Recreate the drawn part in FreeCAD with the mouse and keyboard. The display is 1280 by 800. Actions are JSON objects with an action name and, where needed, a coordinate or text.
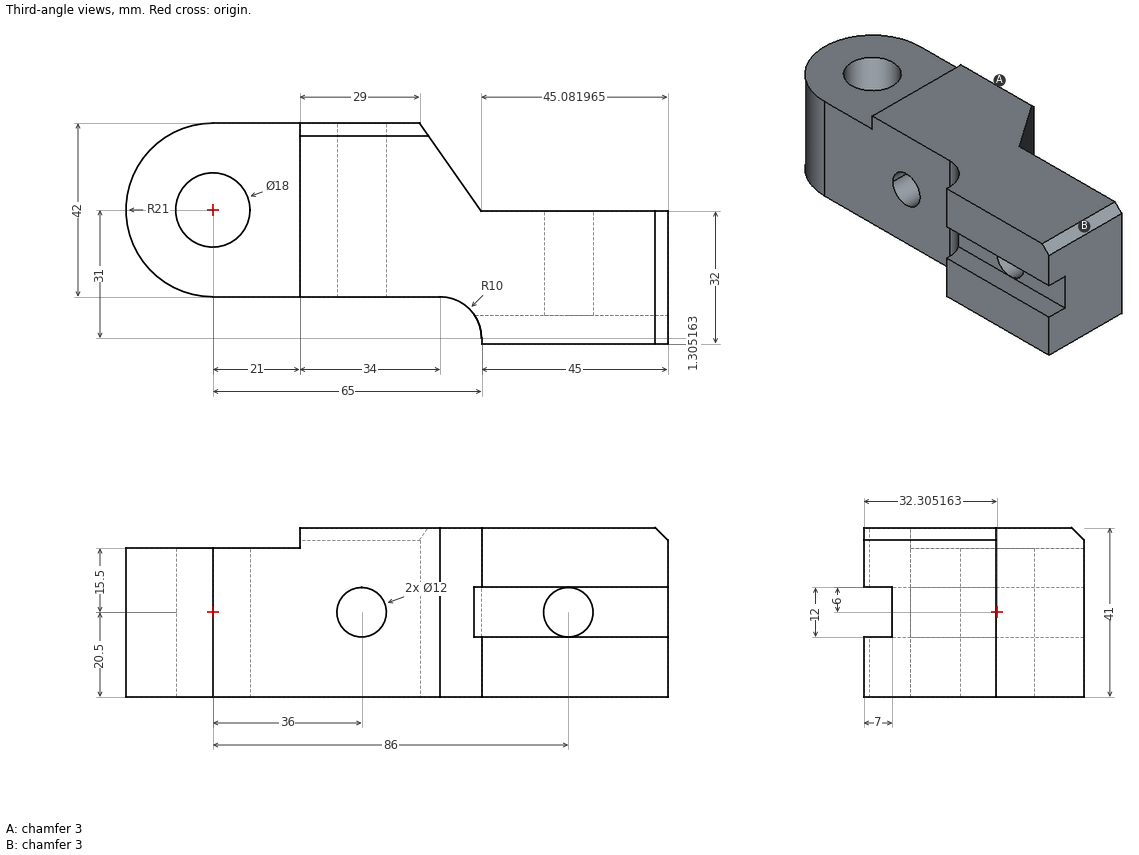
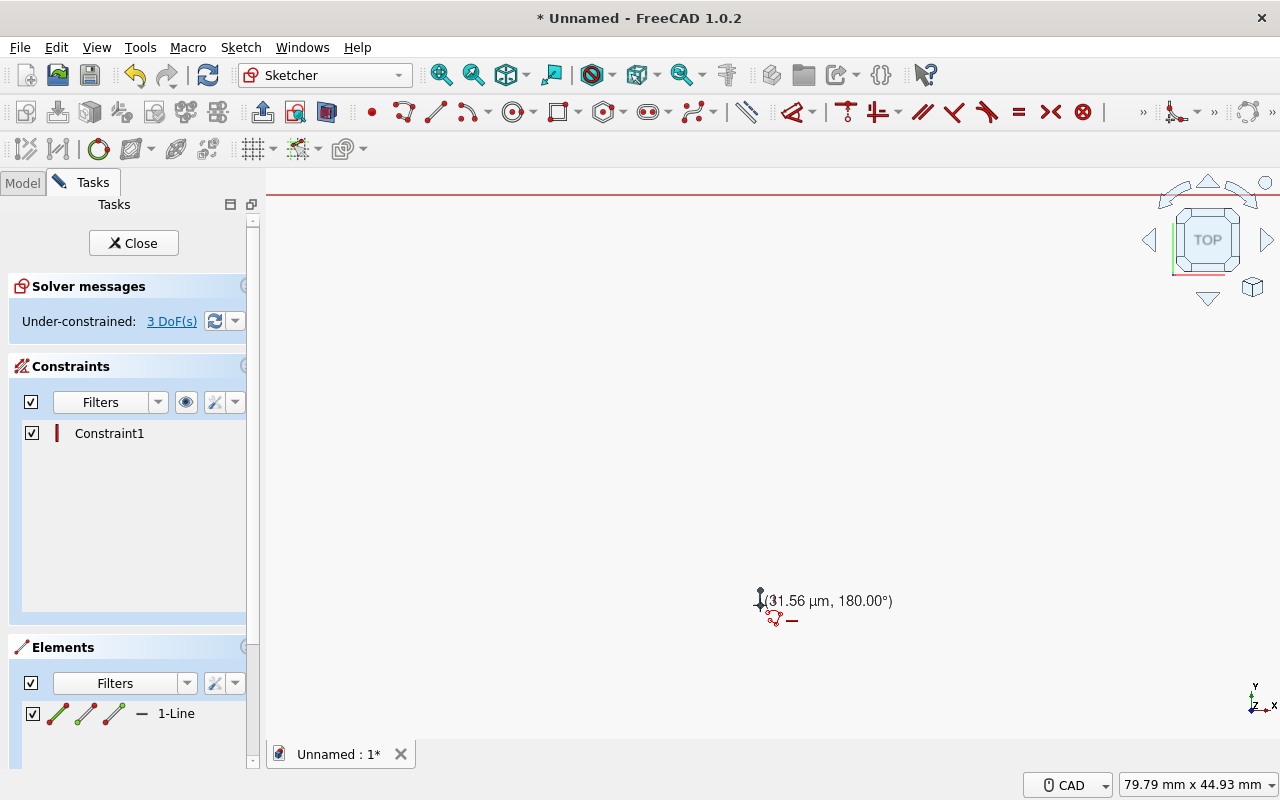
{"action": "scroll", "coordinate": [762, 606], "scroll_direction": "down", "scroll_amount": 4}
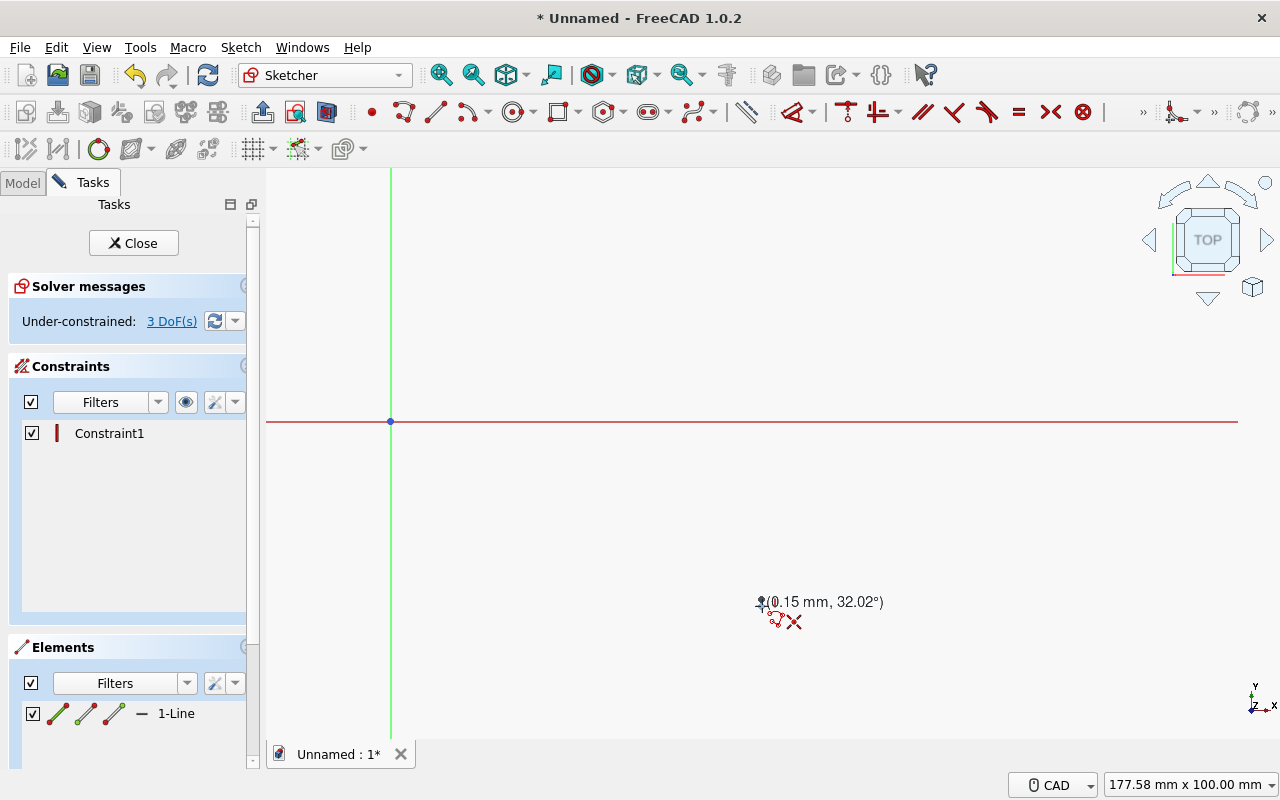
{"action": "left_click", "coordinate": [1019, 606]}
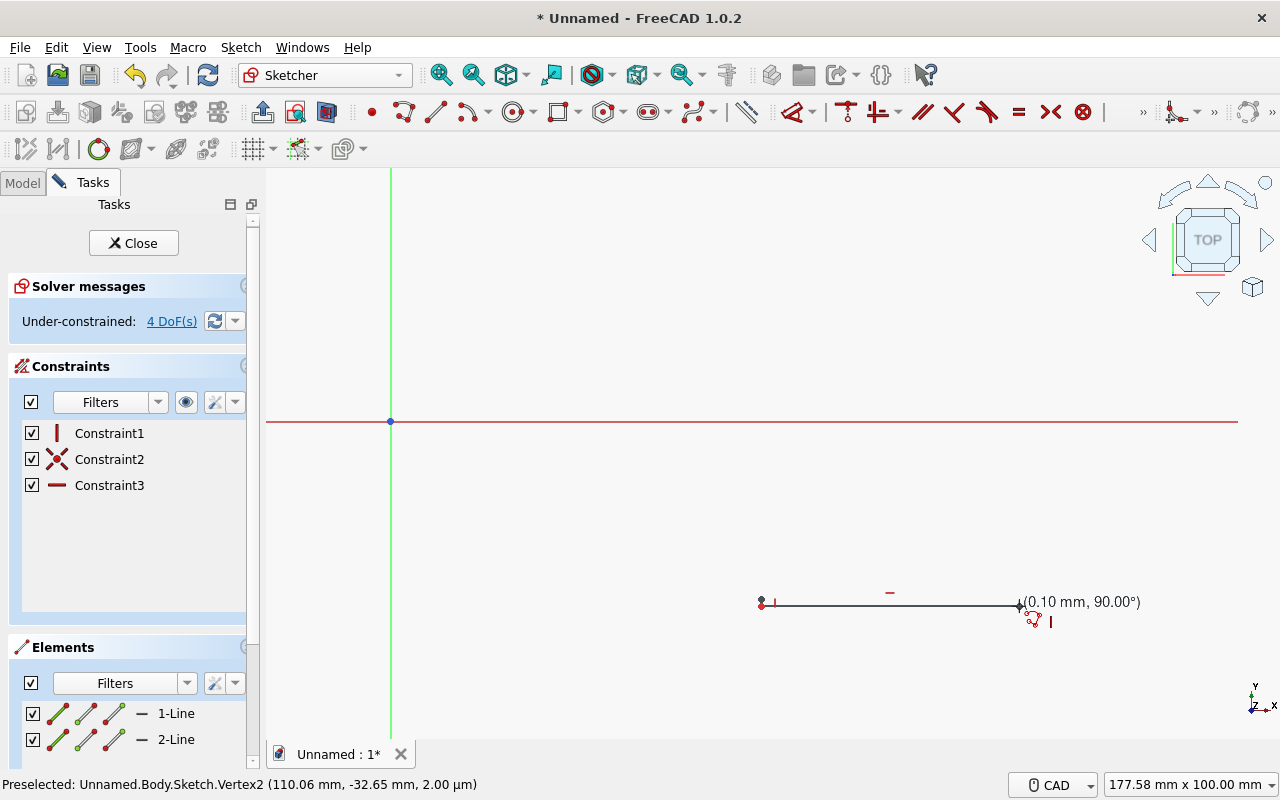
{"action": "scroll", "coordinate": [1019, 423], "scroll_direction": "up", "scroll_amount": 12}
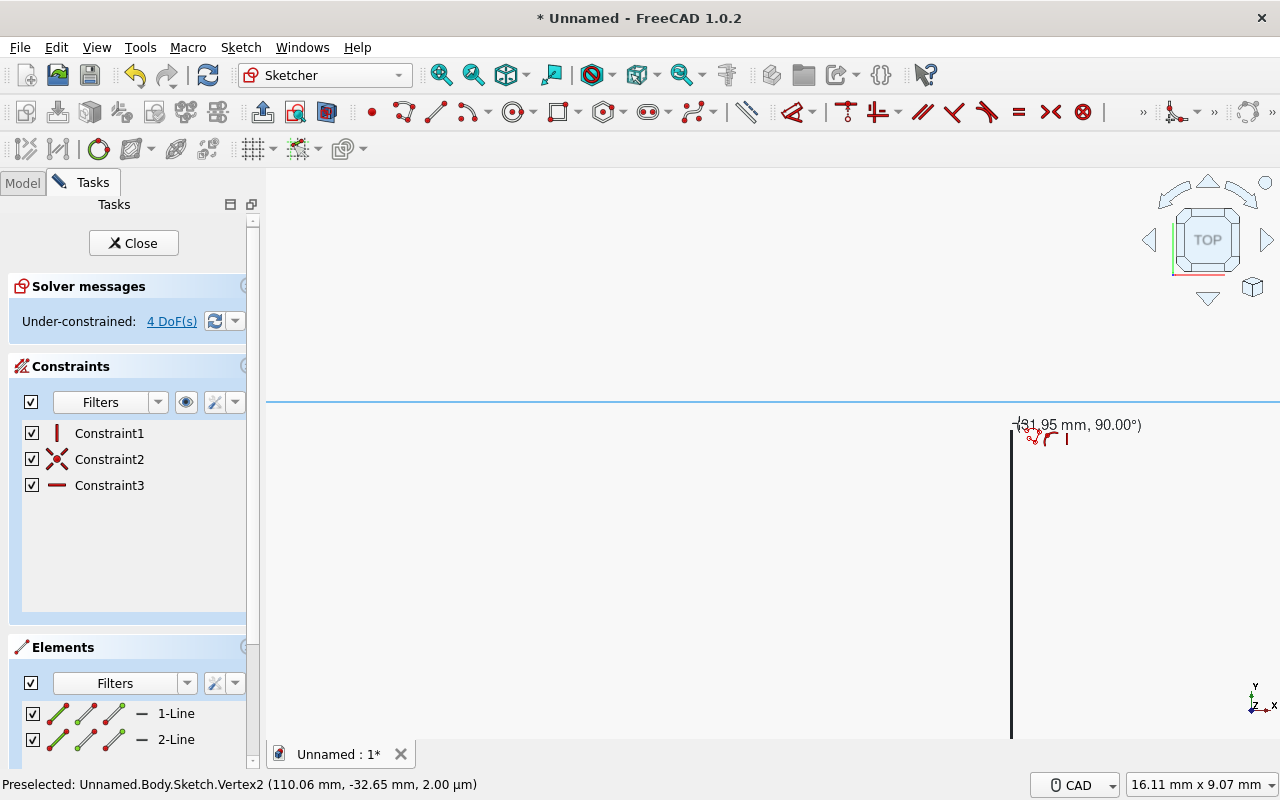
{"action": "left_click", "coordinate": [1012, 422]}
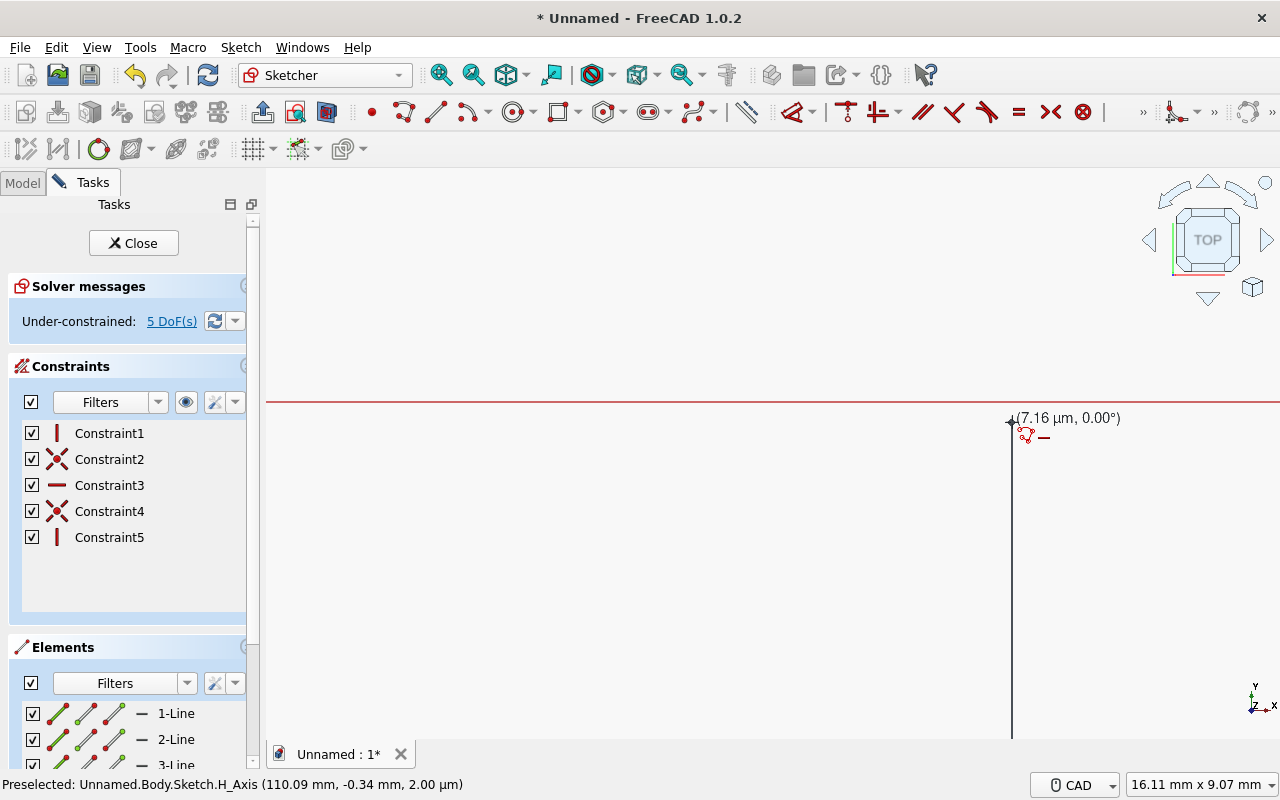
{"action": "scroll", "coordinate": [1020, 423], "scroll_direction": "down", "scroll_amount": 12}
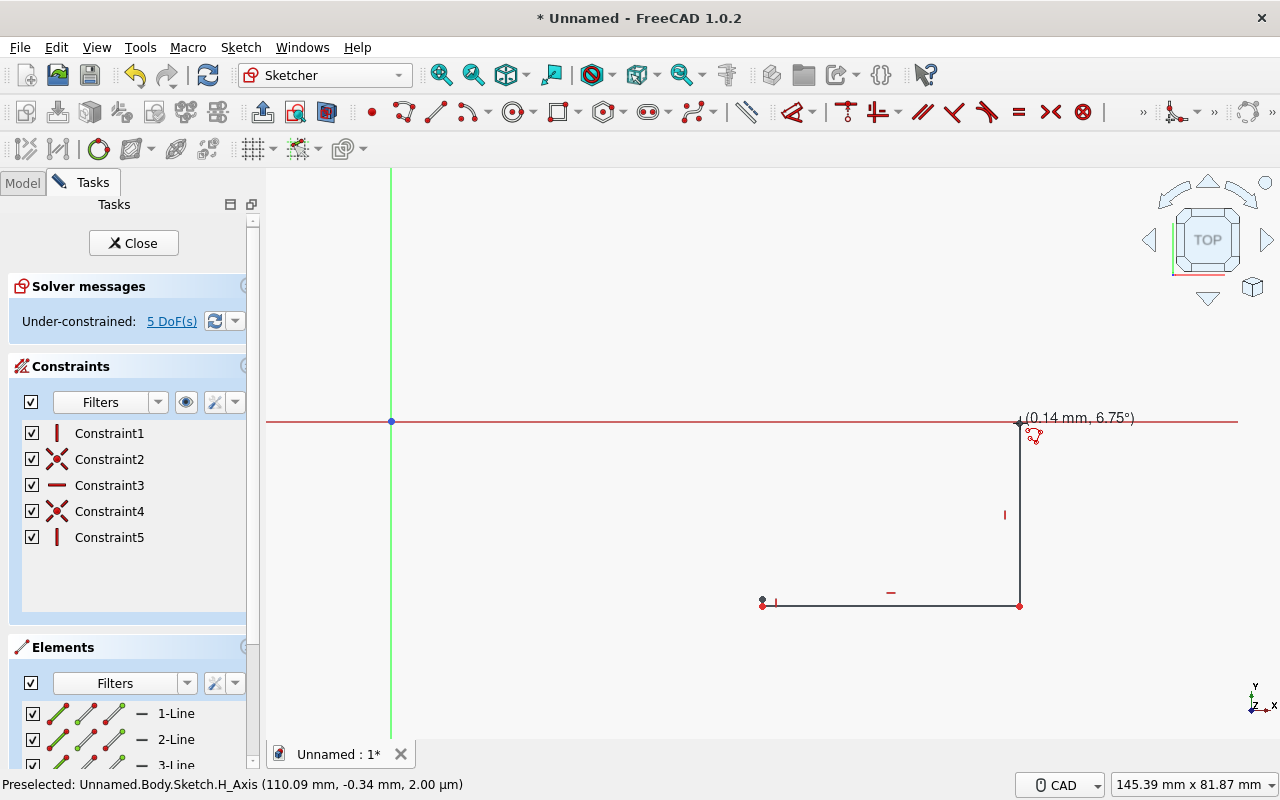
{"action": "scroll", "coordinate": [762, 423], "scroll_direction": "up", "scroll_amount": 12}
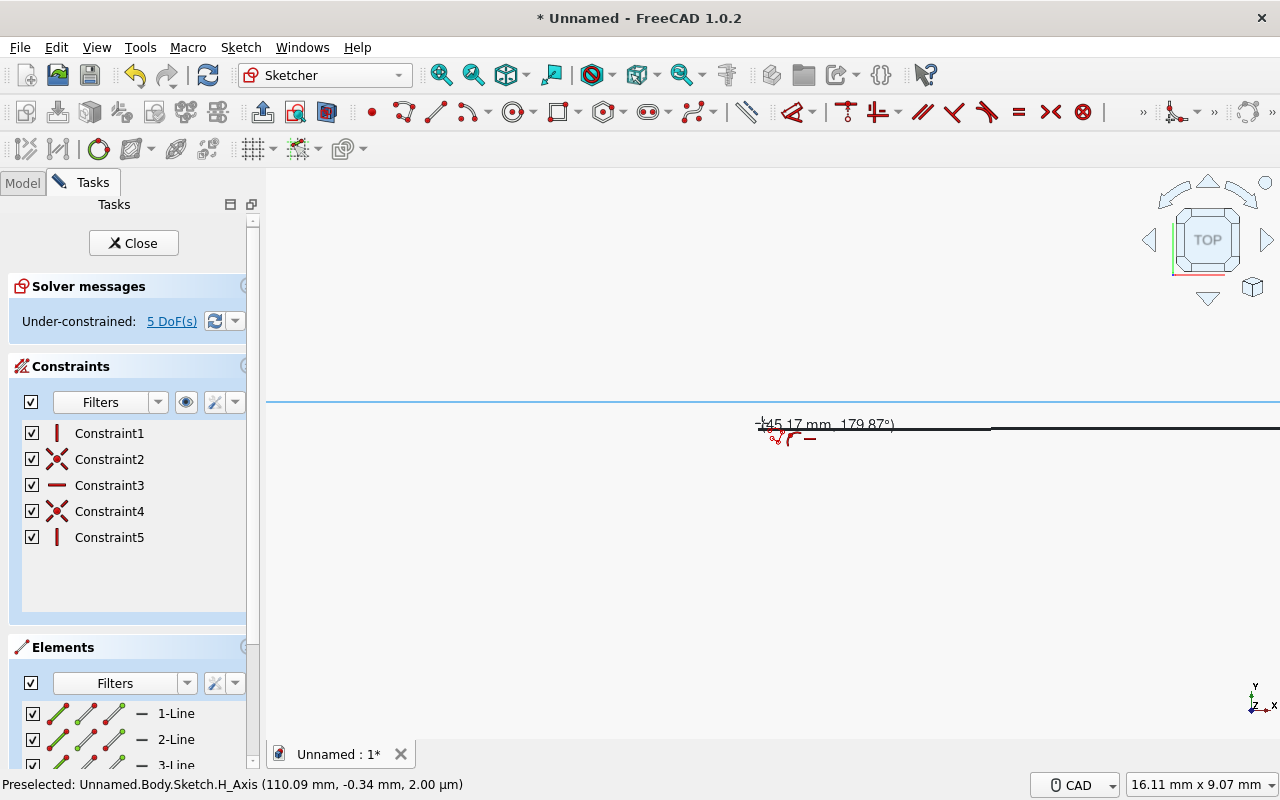
{"action": "left_click", "coordinate": [758, 422]}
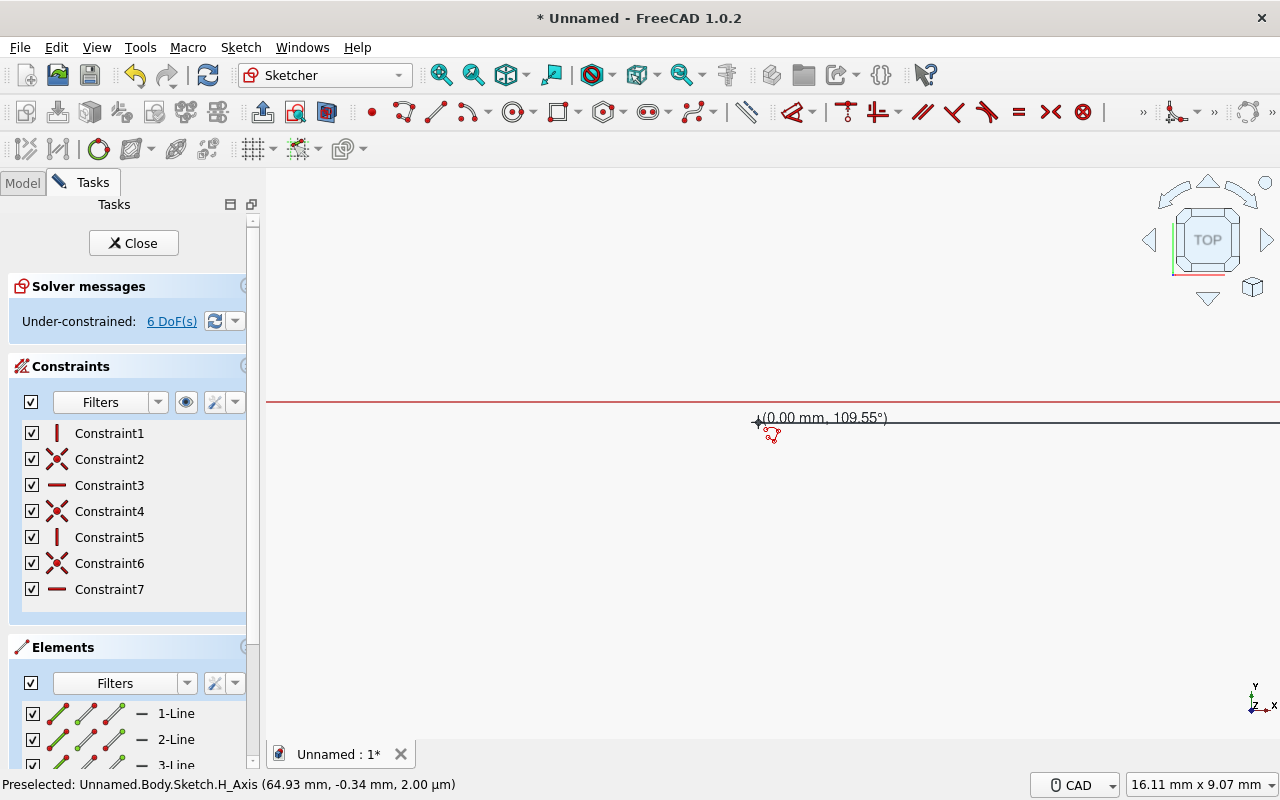
{"action": "scroll", "coordinate": [761, 423], "scroll_direction": "down", "scroll_amount": 12}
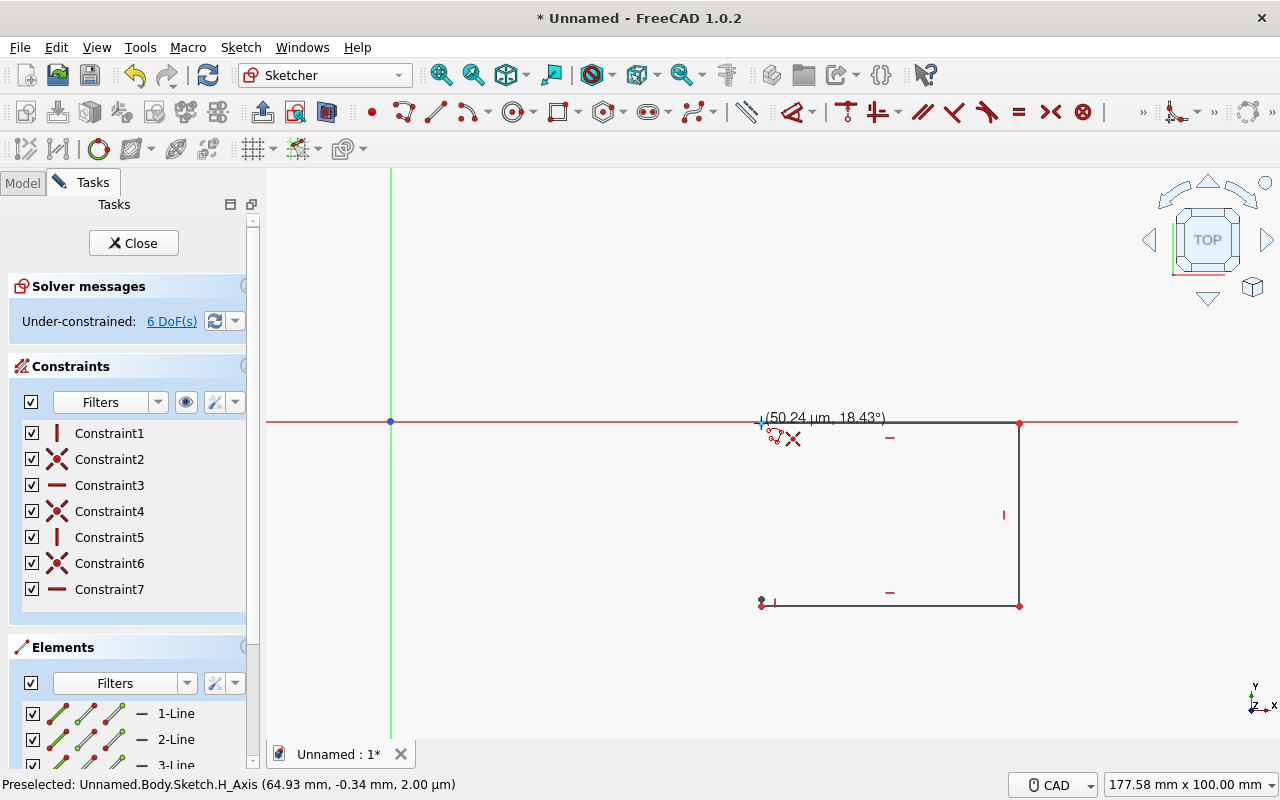
{"action": "left_click", "coordinate": [676, 302]}
{"action": "left_click", "coordinate": [510, 302]}
{"action": "left_click", "coordinate": [510, 541]}
{"action": "left_click", "coordinate": [705, 541]}
{"action": "right_click", "coordinate": [705, 541]}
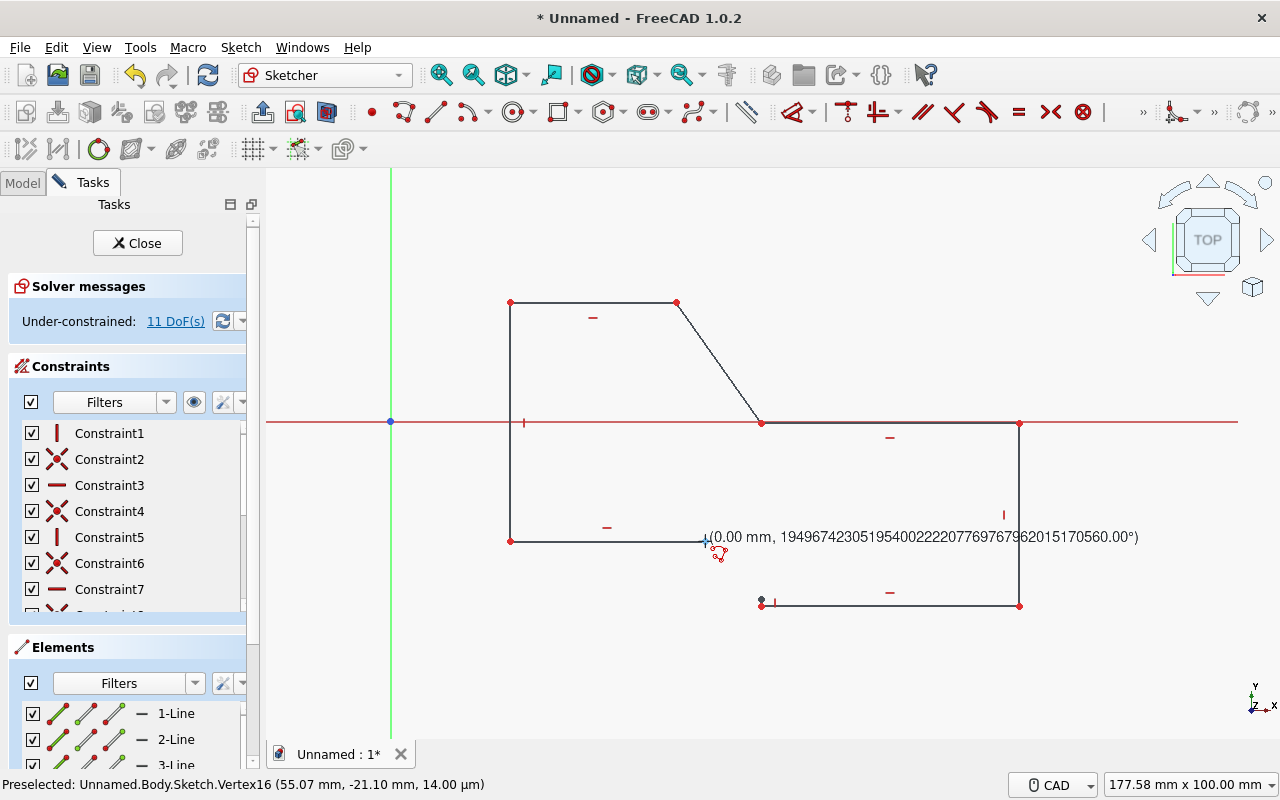
{"action": "left_click", "coordinate": [490, 112]}